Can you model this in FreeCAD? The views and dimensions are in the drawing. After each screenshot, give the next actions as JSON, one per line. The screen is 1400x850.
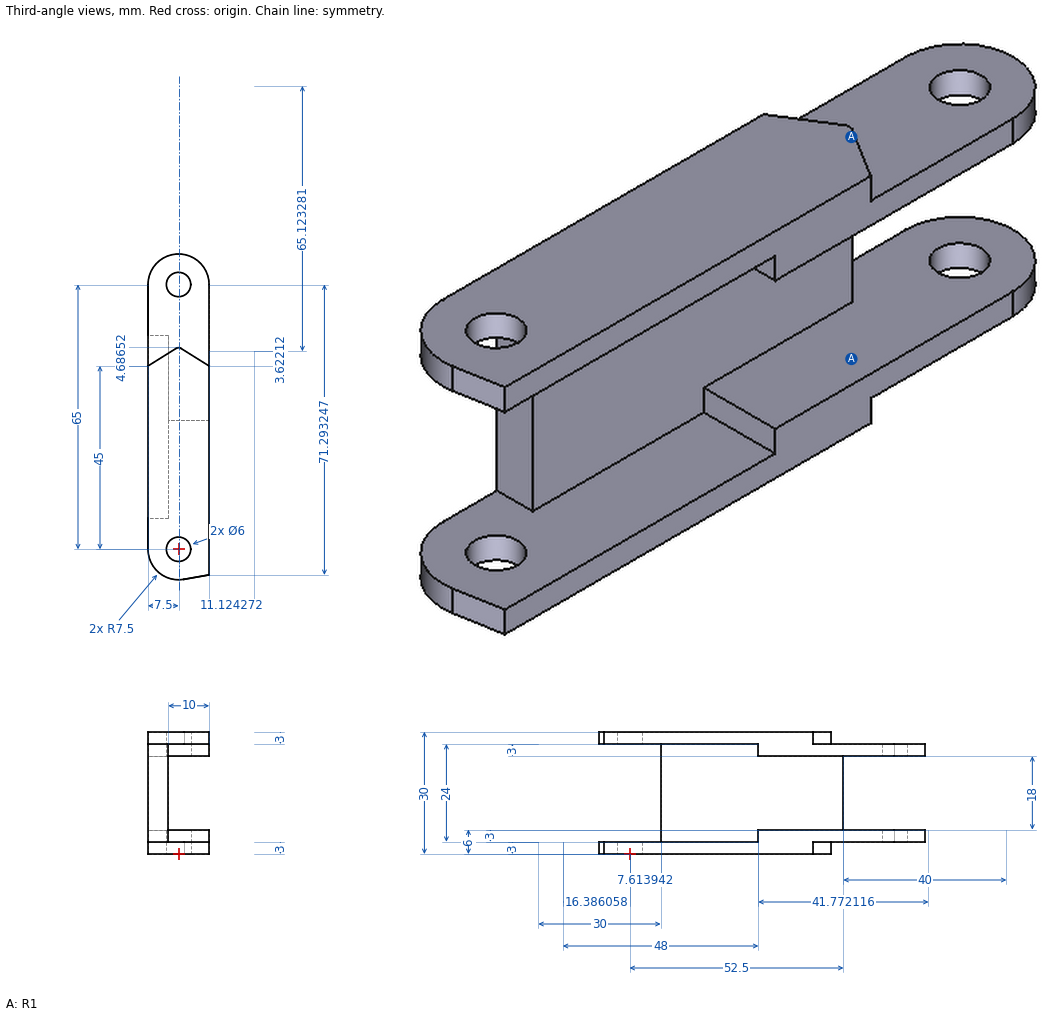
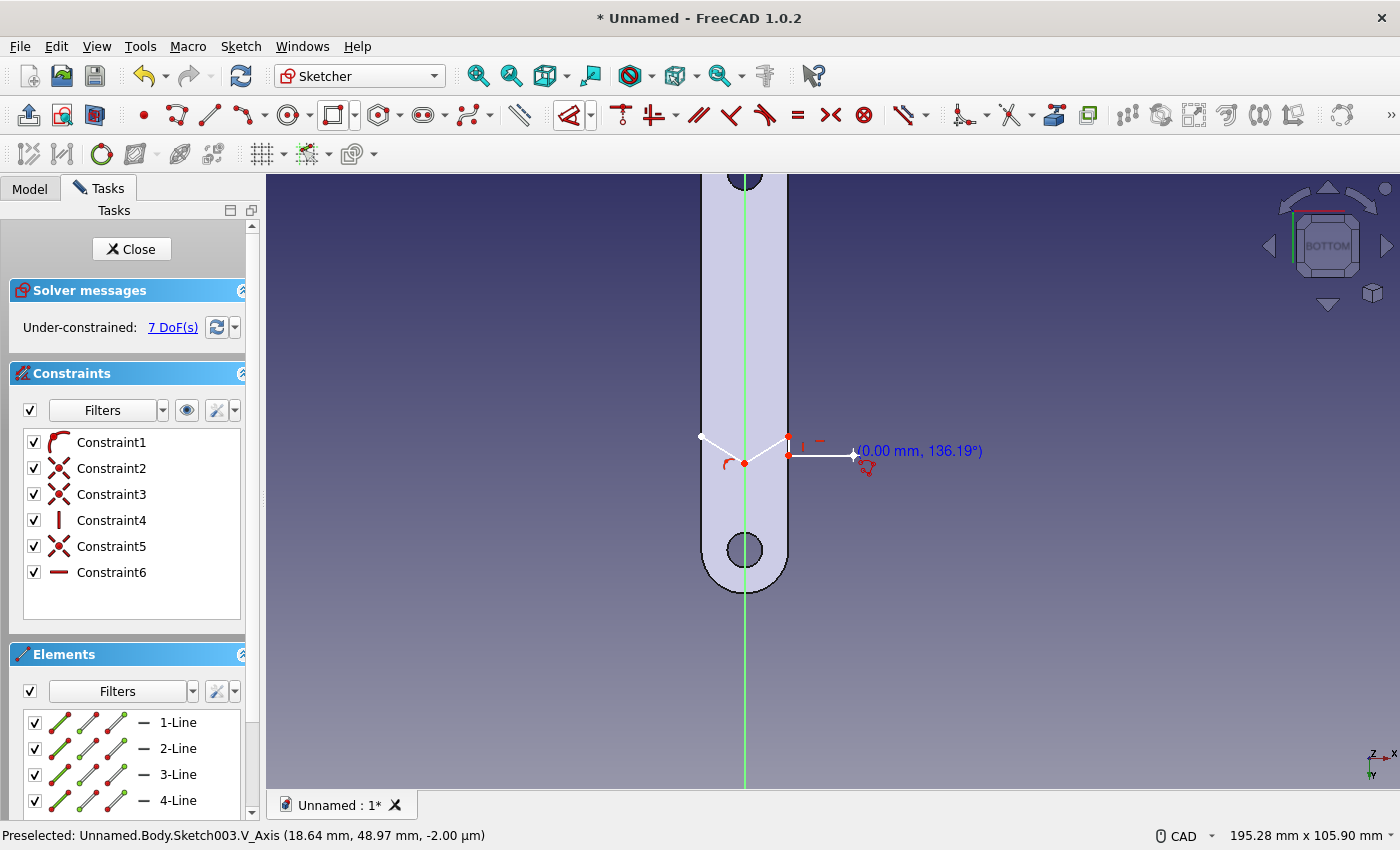
{"action": "scroll", "coordinate": [789, 456], "scroll_direction": "down", "scroll_amount": 3}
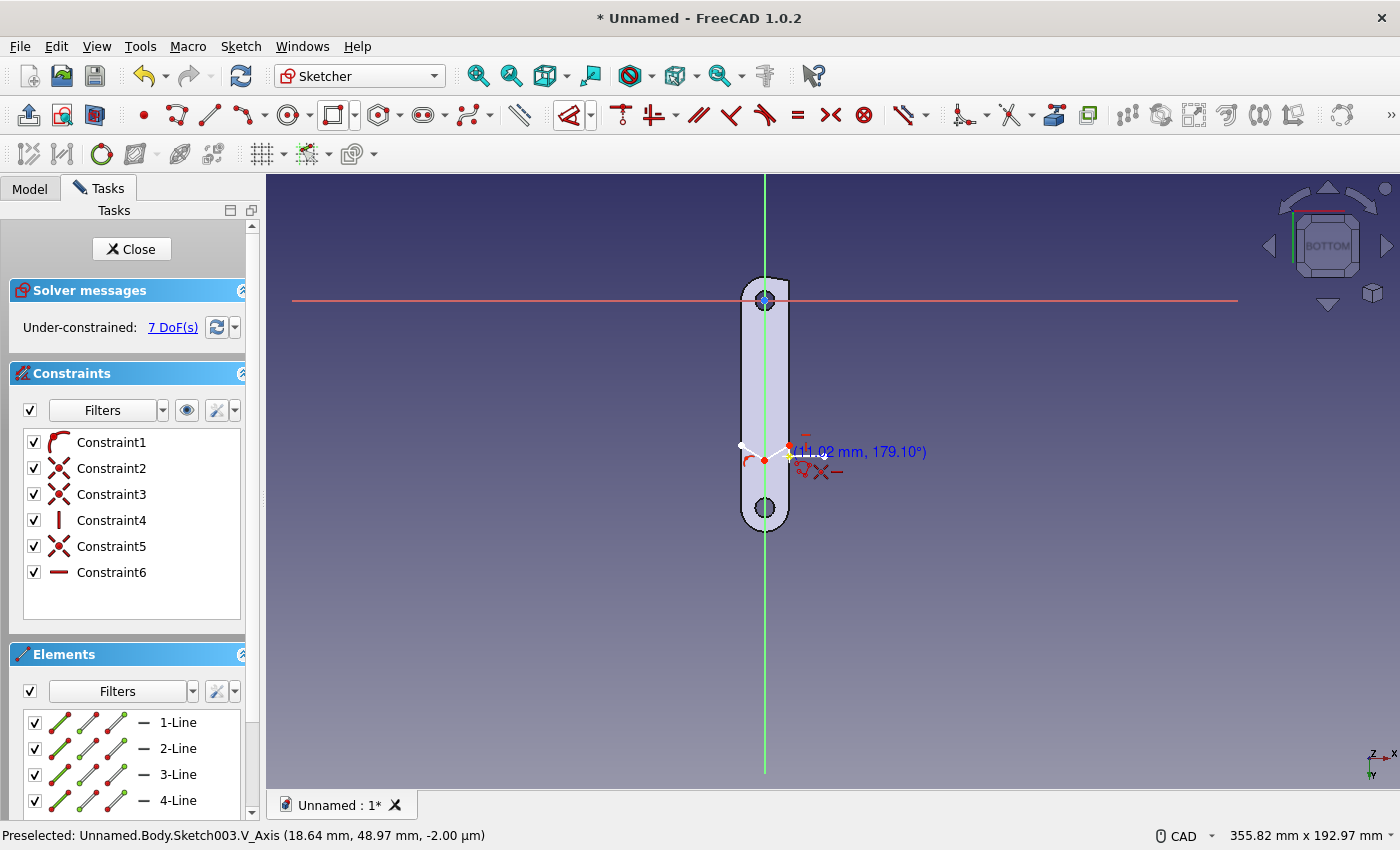
{"action": "left_click", "coordinate": [824, 663]}
{"action": "left_click", "coordinate": [706, 663]}
{"action": "left_click", "coordinate": [706, 456]}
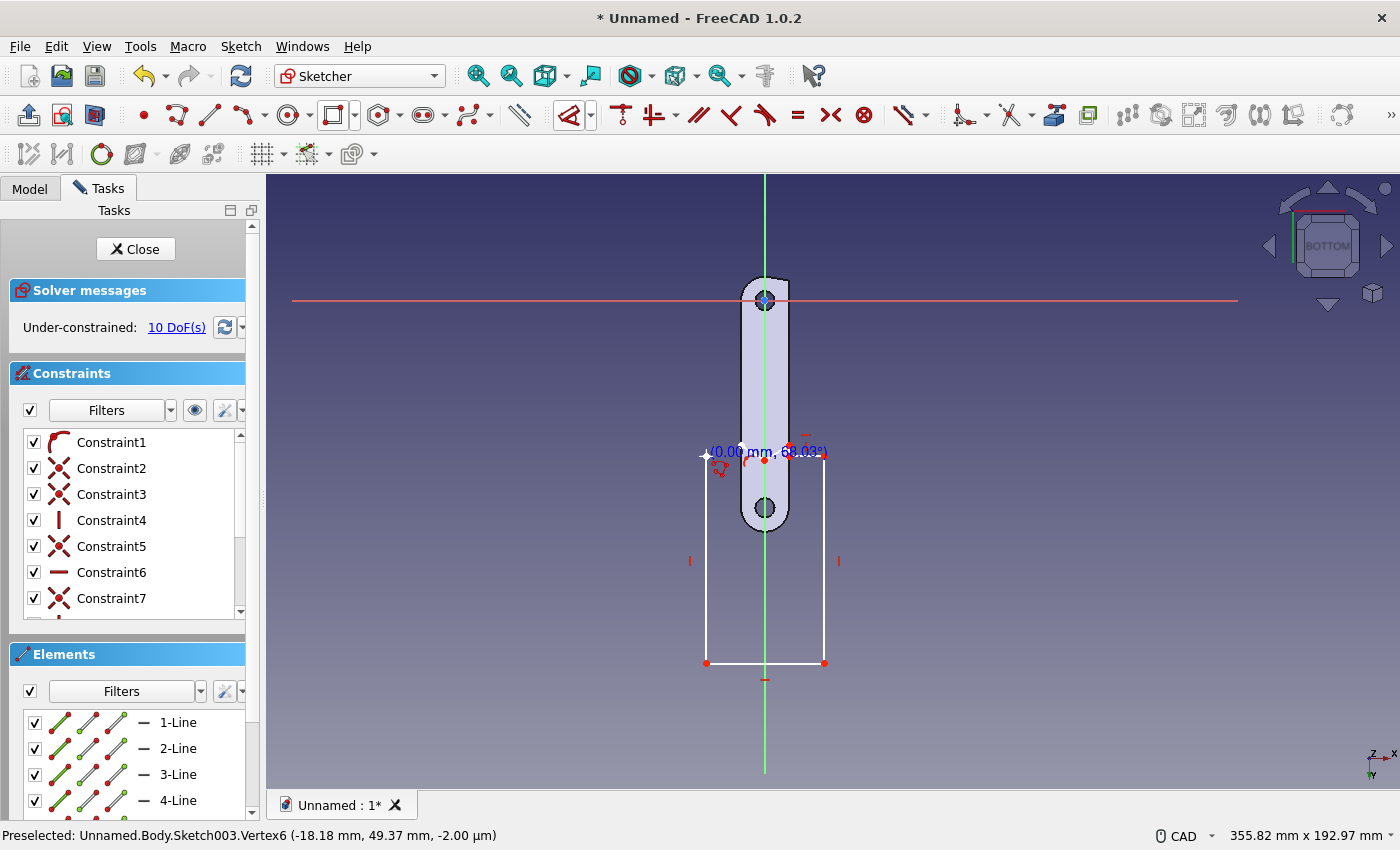
{"action": "scroll", "coordinate": [741, 456], "scroll_direction": "up", "scroll_amount": 3}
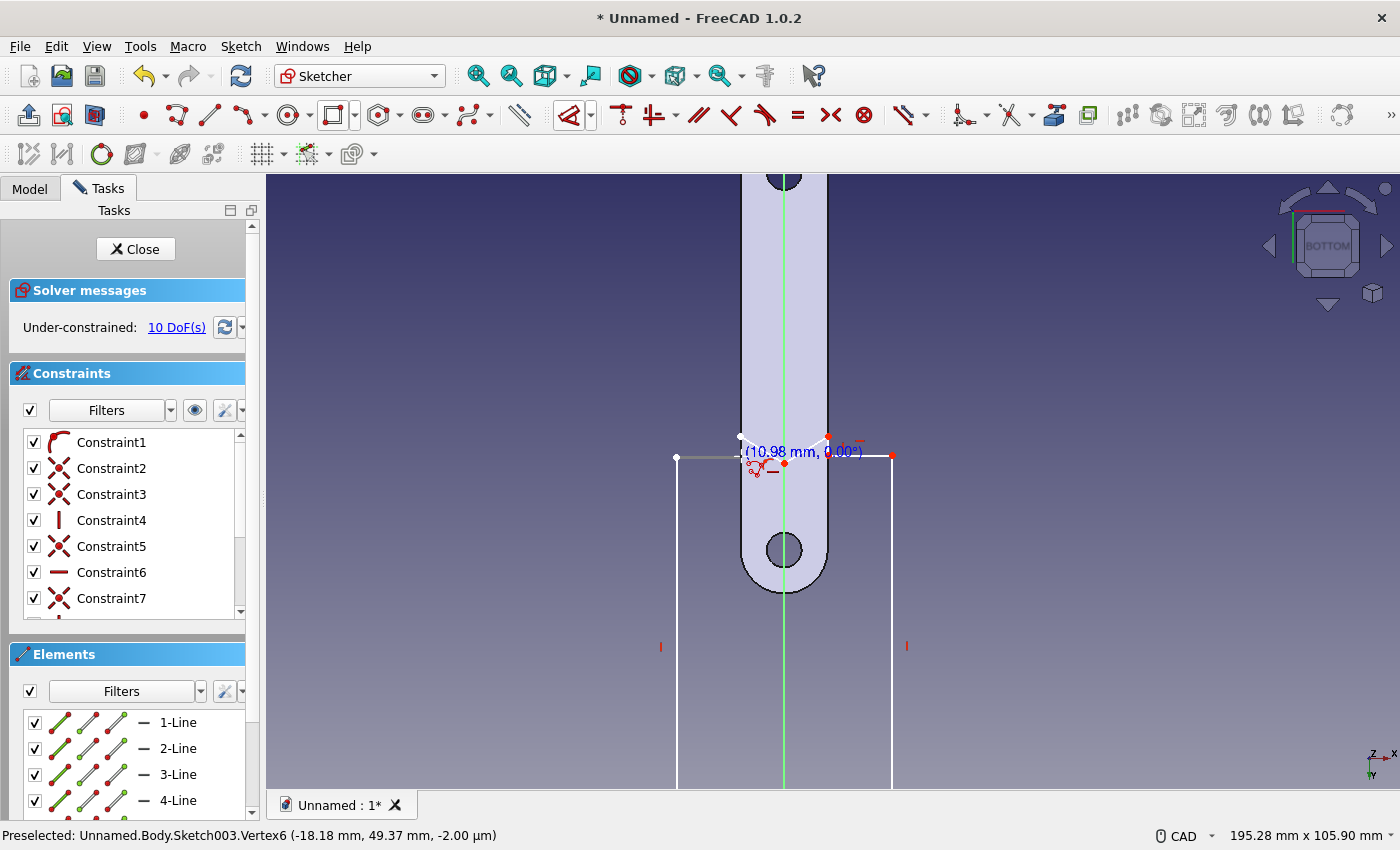
{"action": "left_click", "coordinate": [741, 456]}
{"action": "left_click", "coordinate": [741, 436]}
{"action": "key", "text": "Escape"}
{"action": "key", "text": "Escape"}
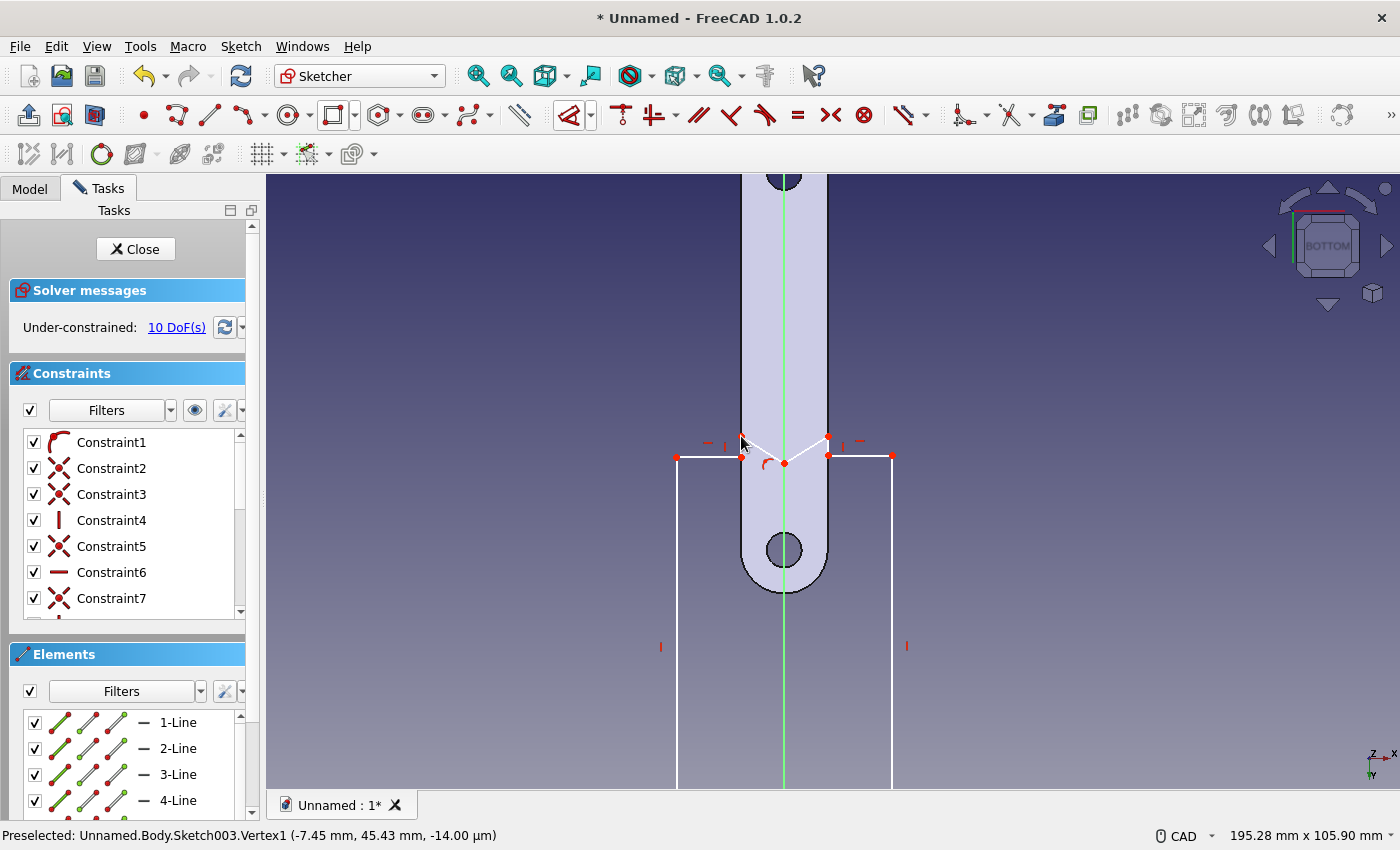
{"action": "left_click", "coordinate": [741, 436]}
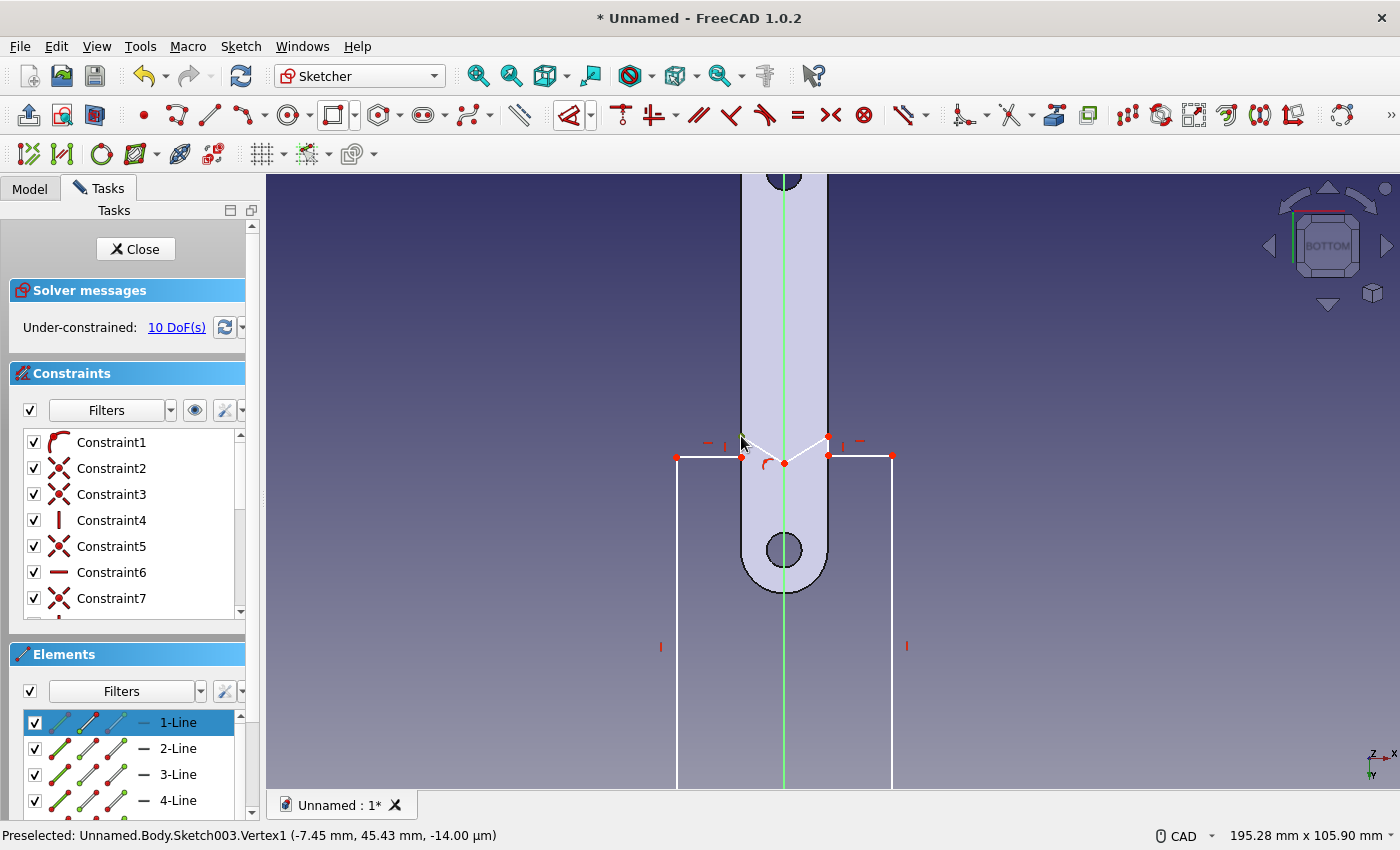
{"action": "left_click", "coordinate": [828, 436]}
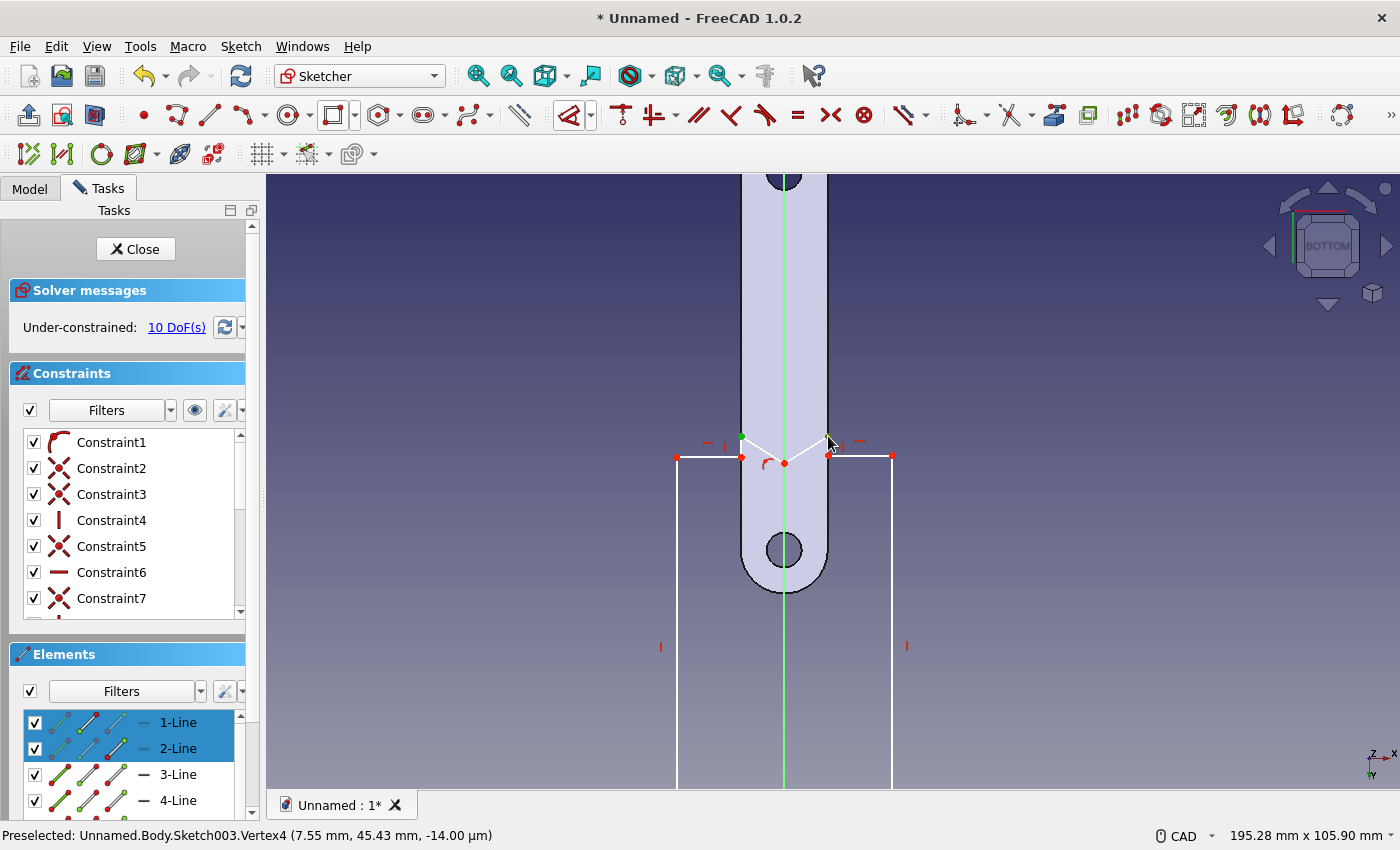
{"action": "left_click", "coordinate": [784, 721]}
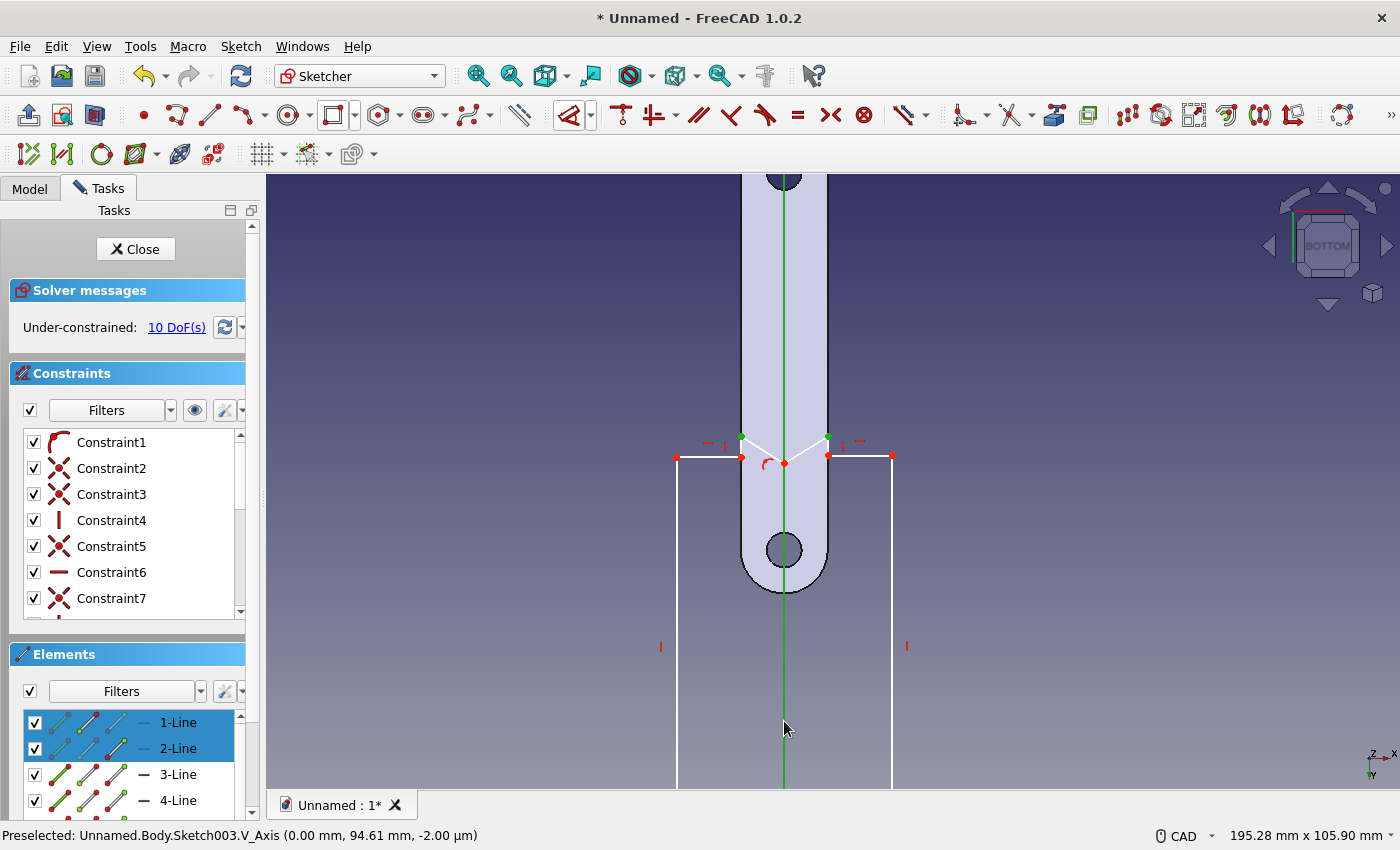
{"action": "key", "text": "s"}